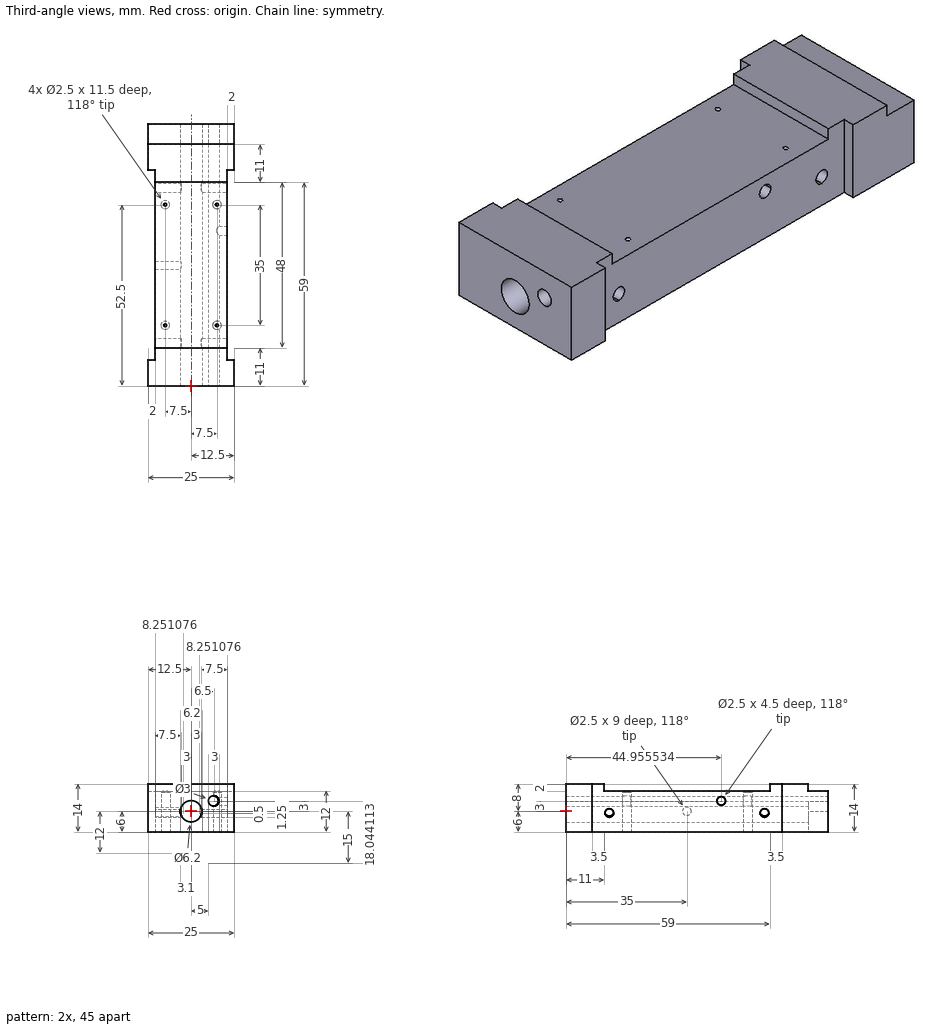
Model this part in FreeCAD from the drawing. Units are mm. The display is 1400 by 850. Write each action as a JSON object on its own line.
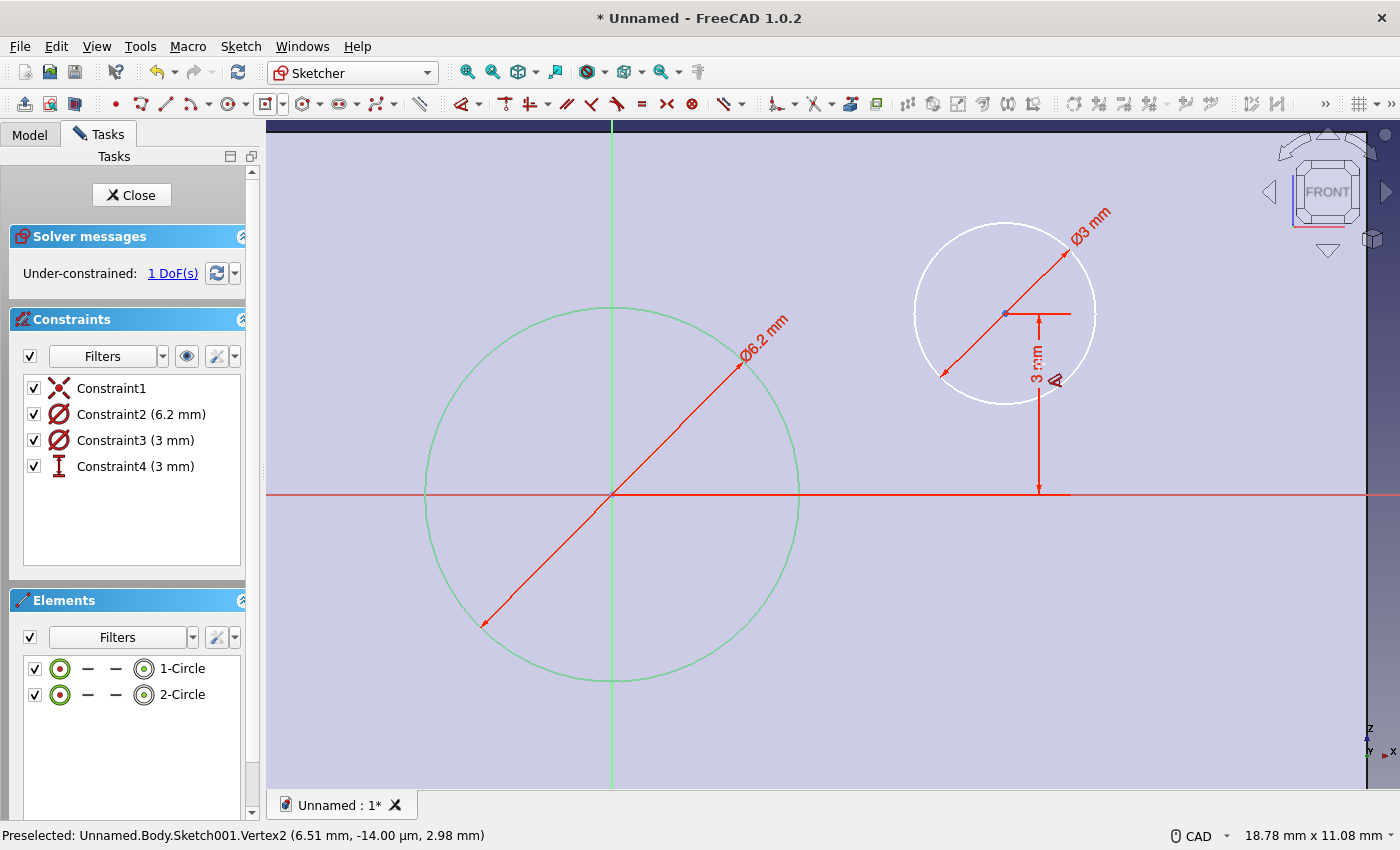
{"action": "left_click", "coordinate": [1005, 314]}
{"action": "left_click", "coordinate": [809, 280]}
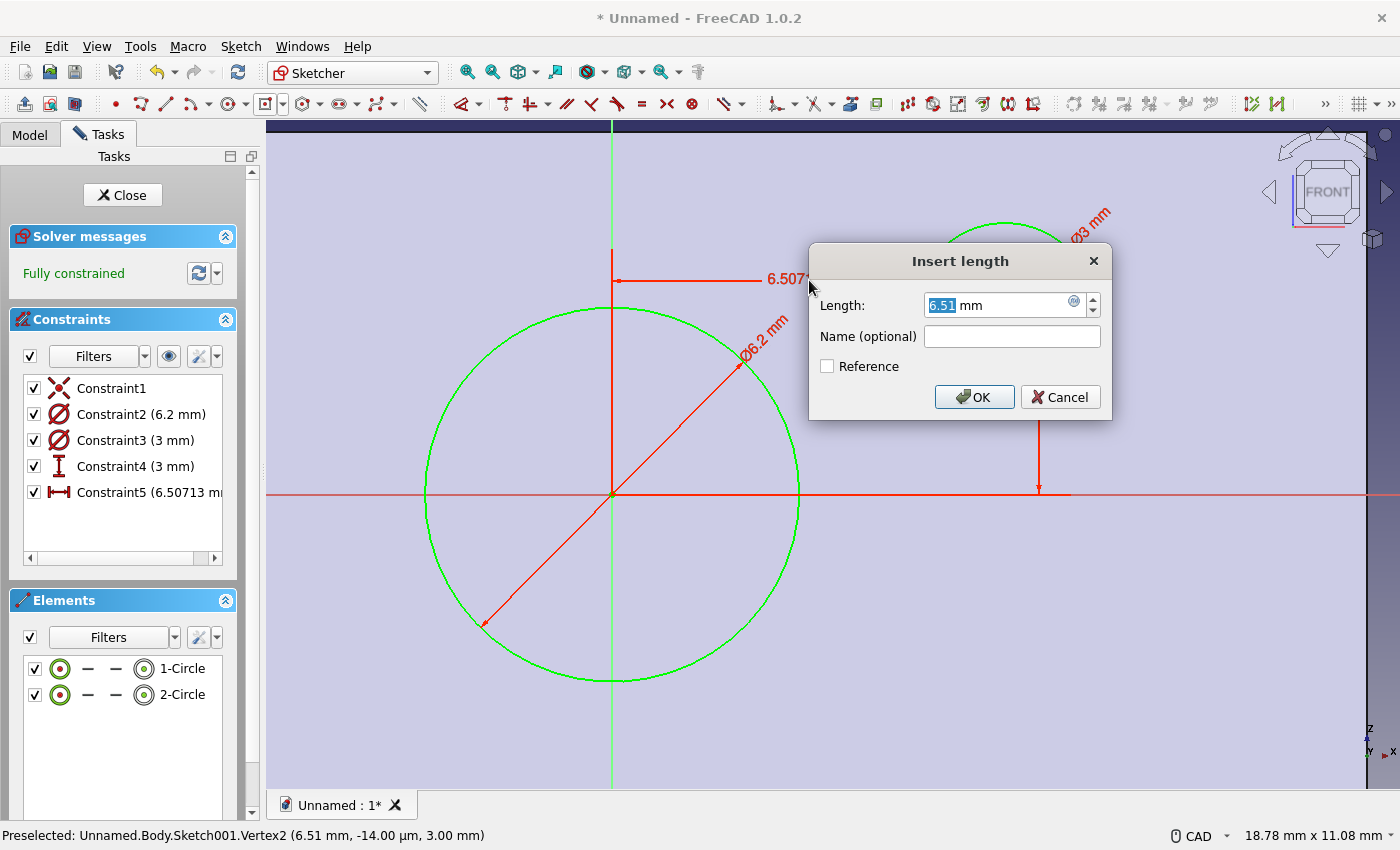
{"action": "type", "text": "6.5"}
{"action": "key", "text": "Return"}
{"action": "key", "text": "Escape"}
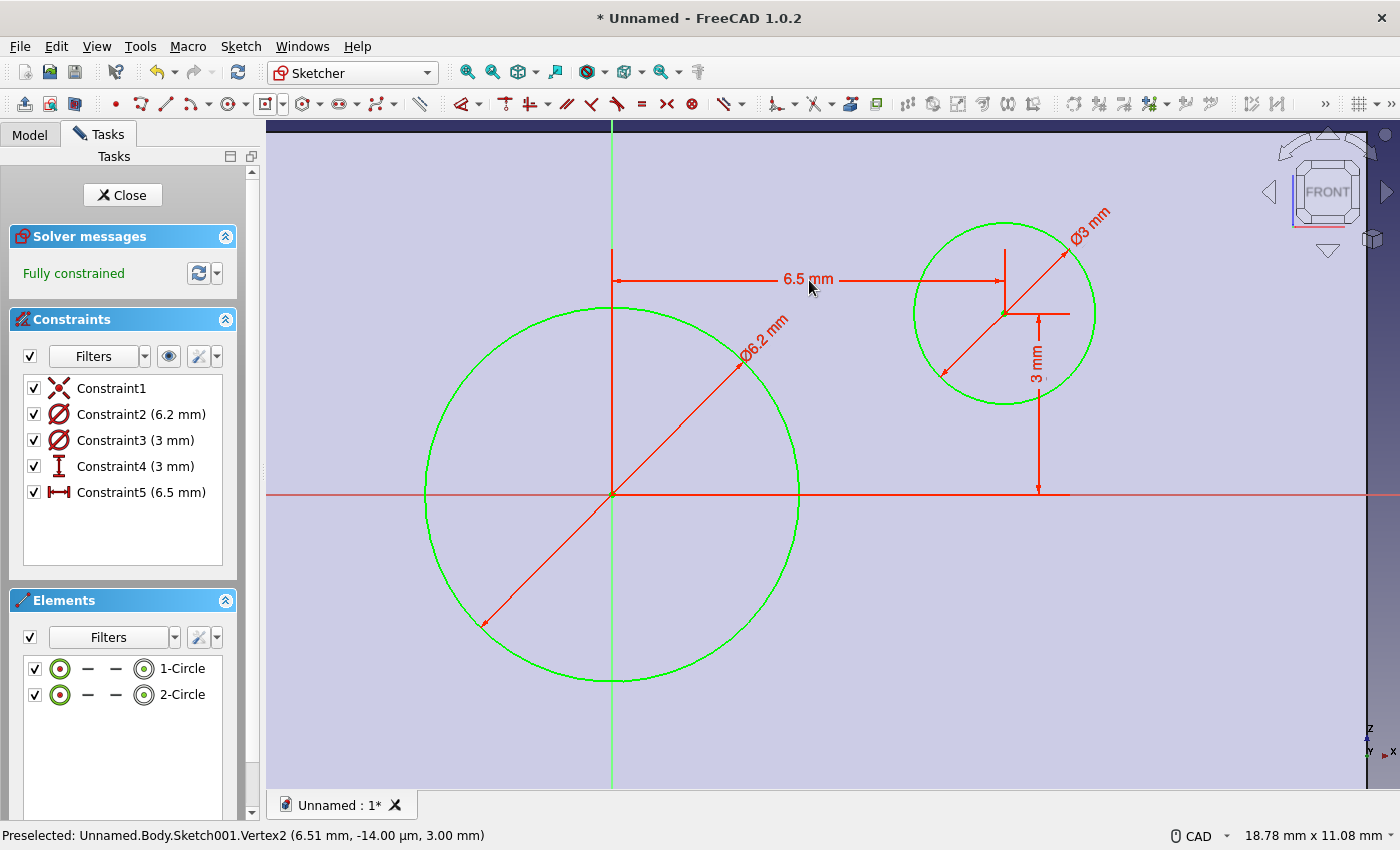
{"action": "left_click", "coordinate": [123, 195]}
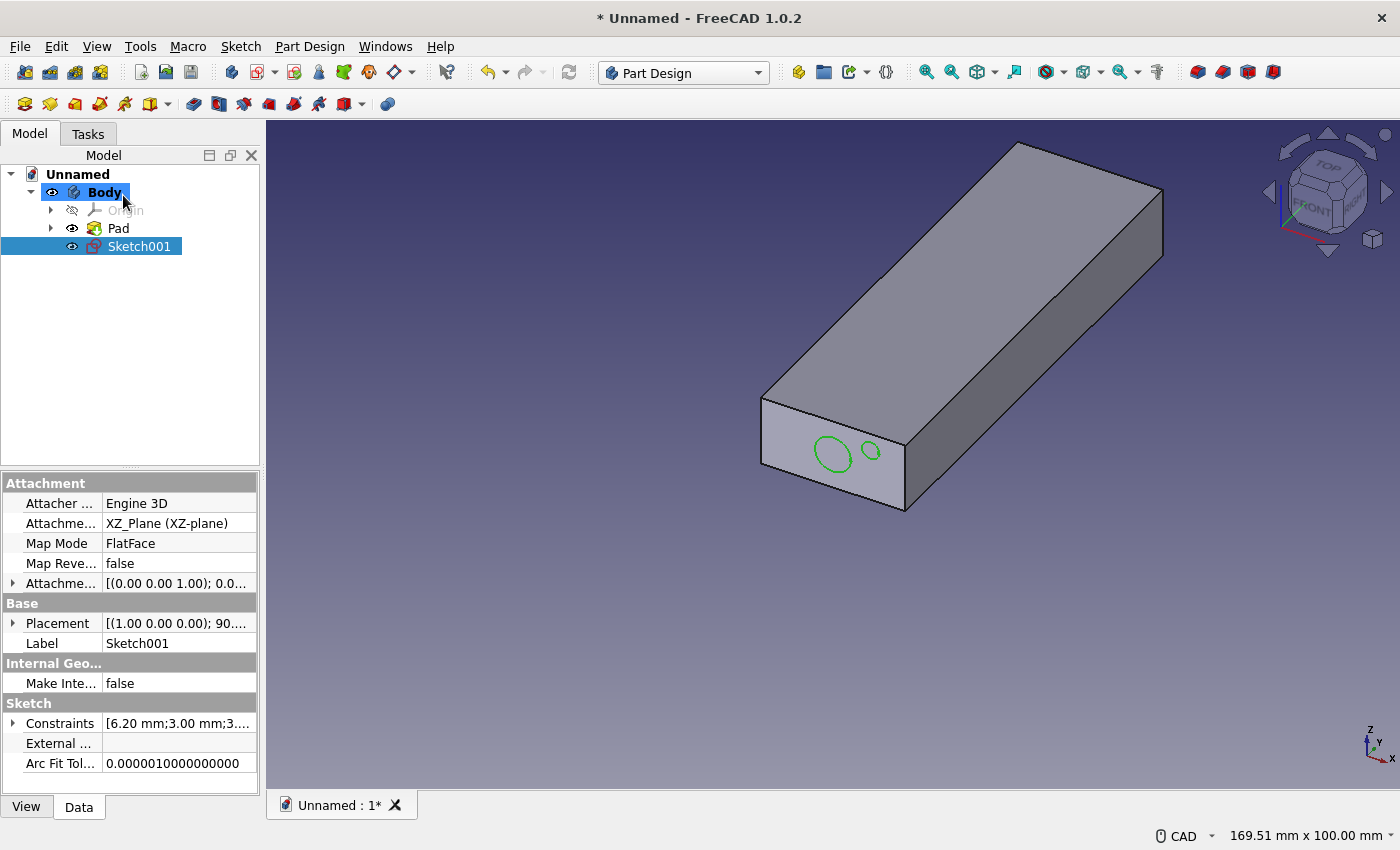
{"action": "left_click", "coordinate": [194, 104]}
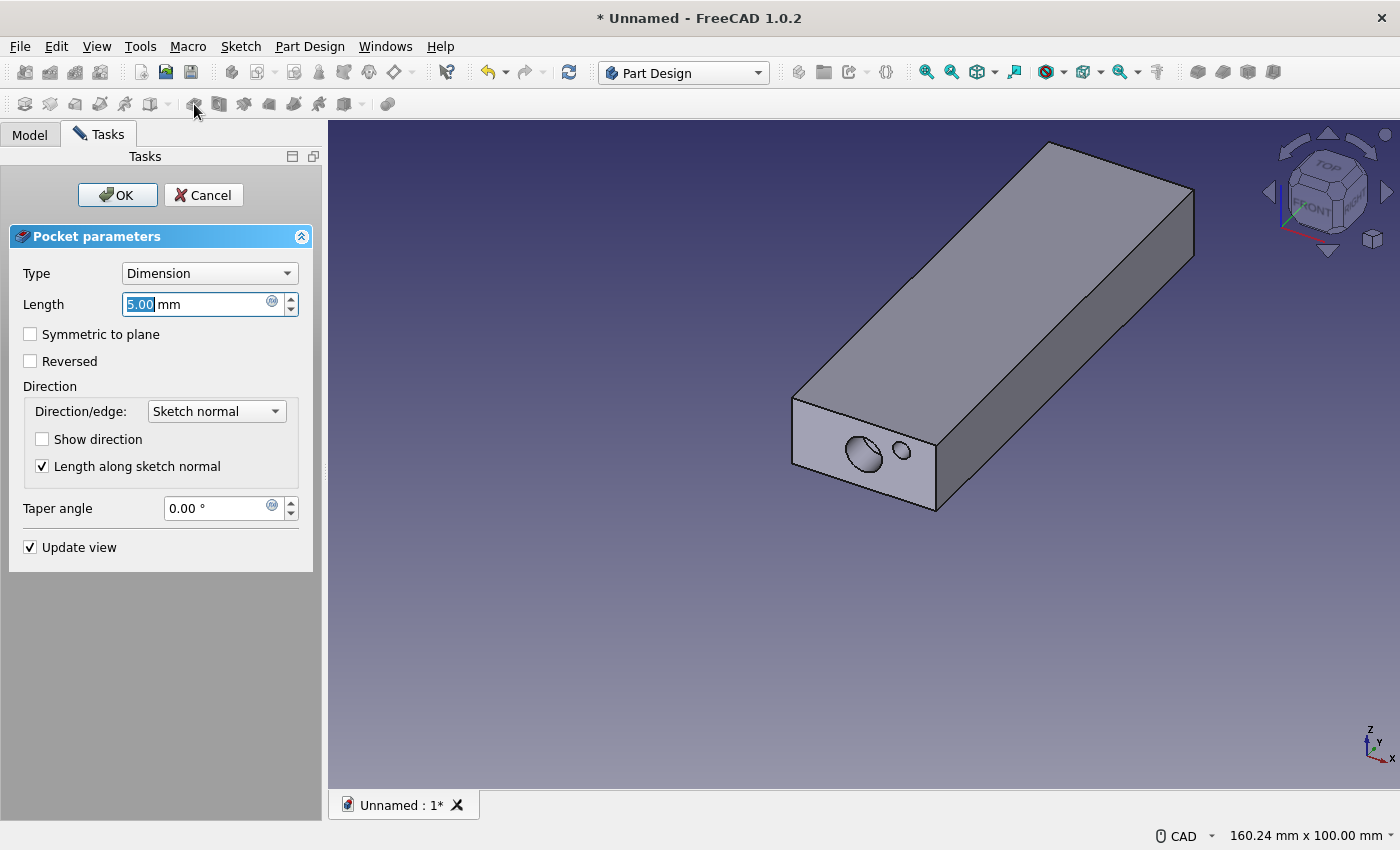
{"action": "left_click", "coordinate": [210, 274]}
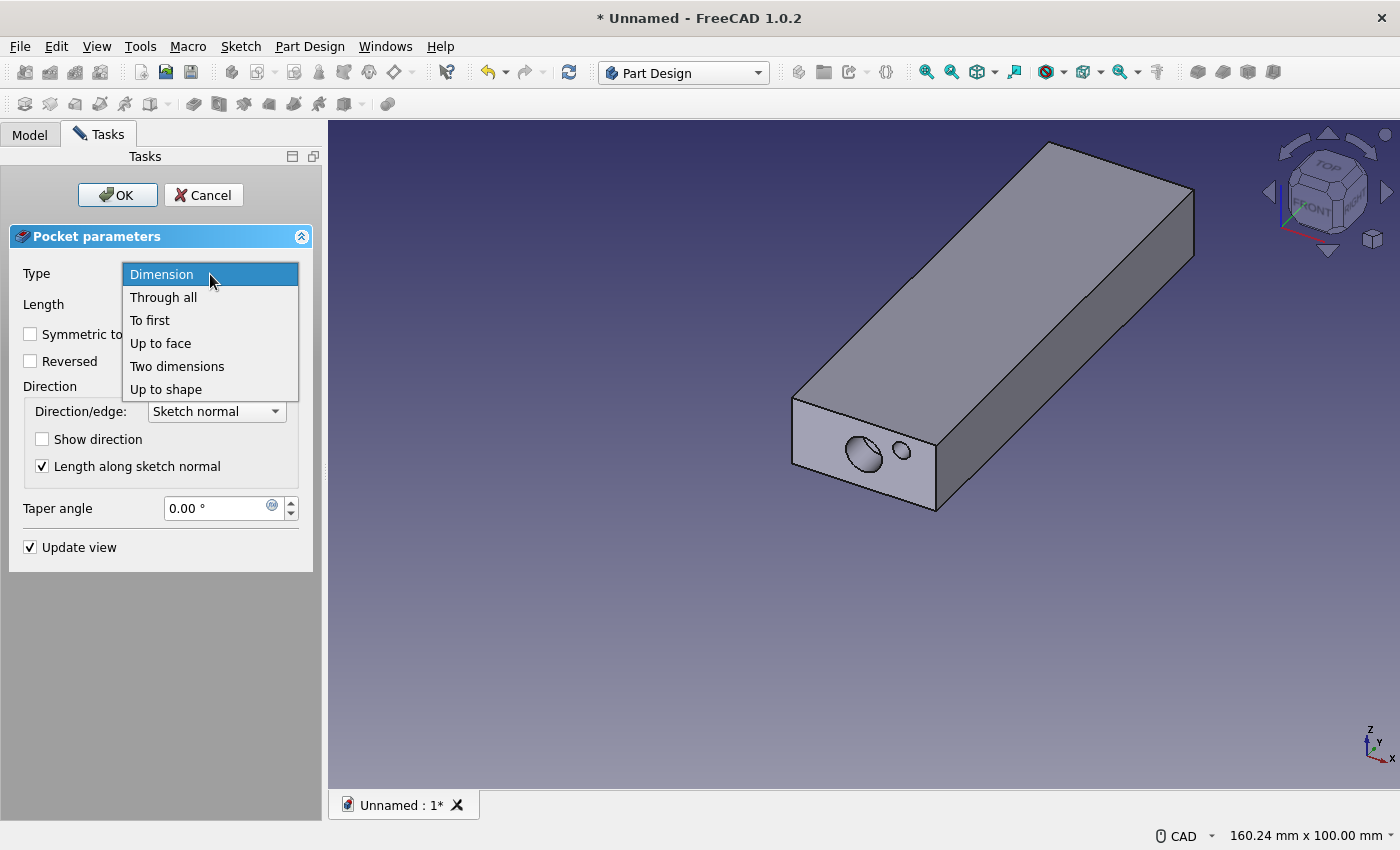
{"action": "left_click", "coordinate": [208, 298]}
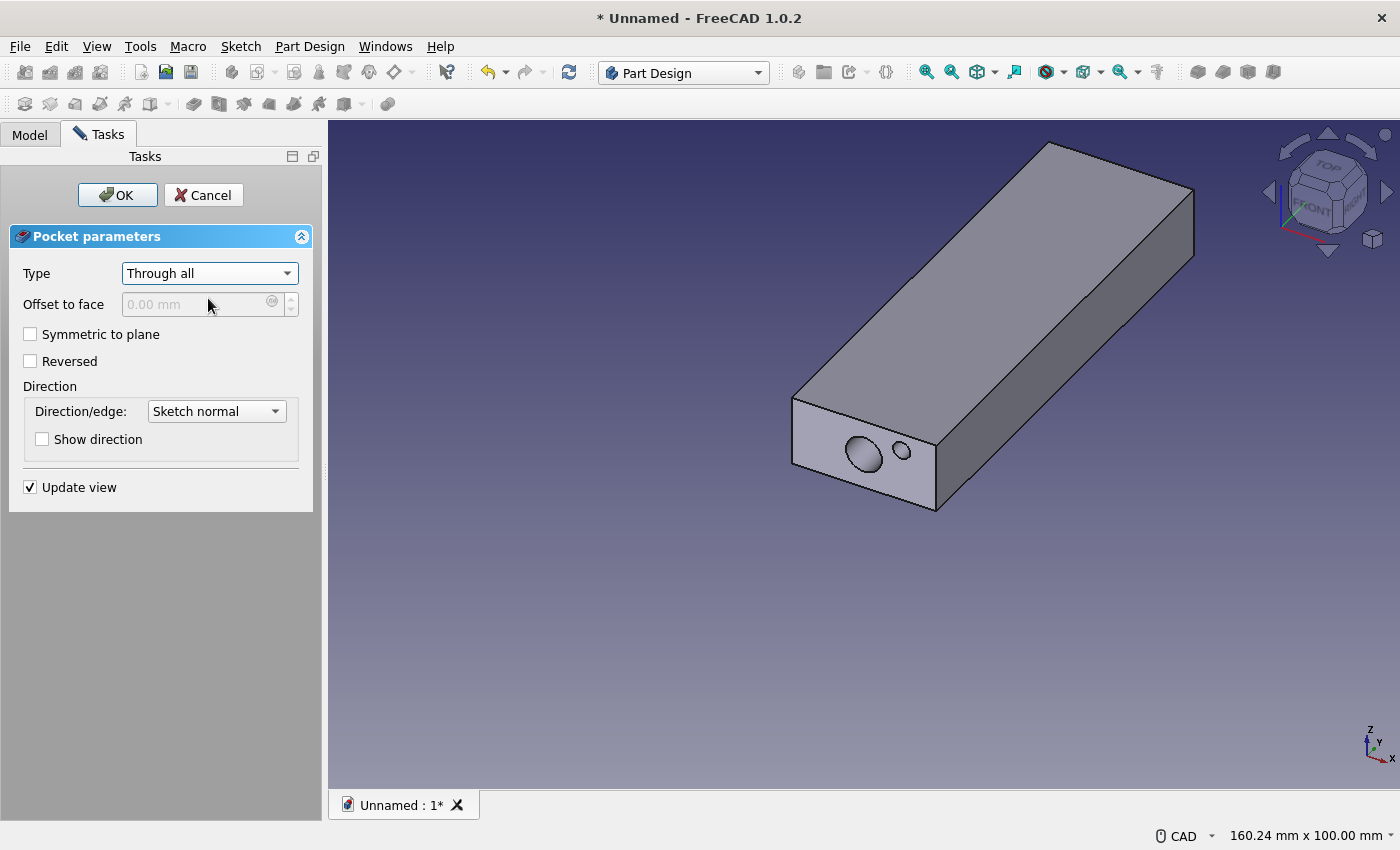
{"action": "left_click", "coordinate": [118, 195]}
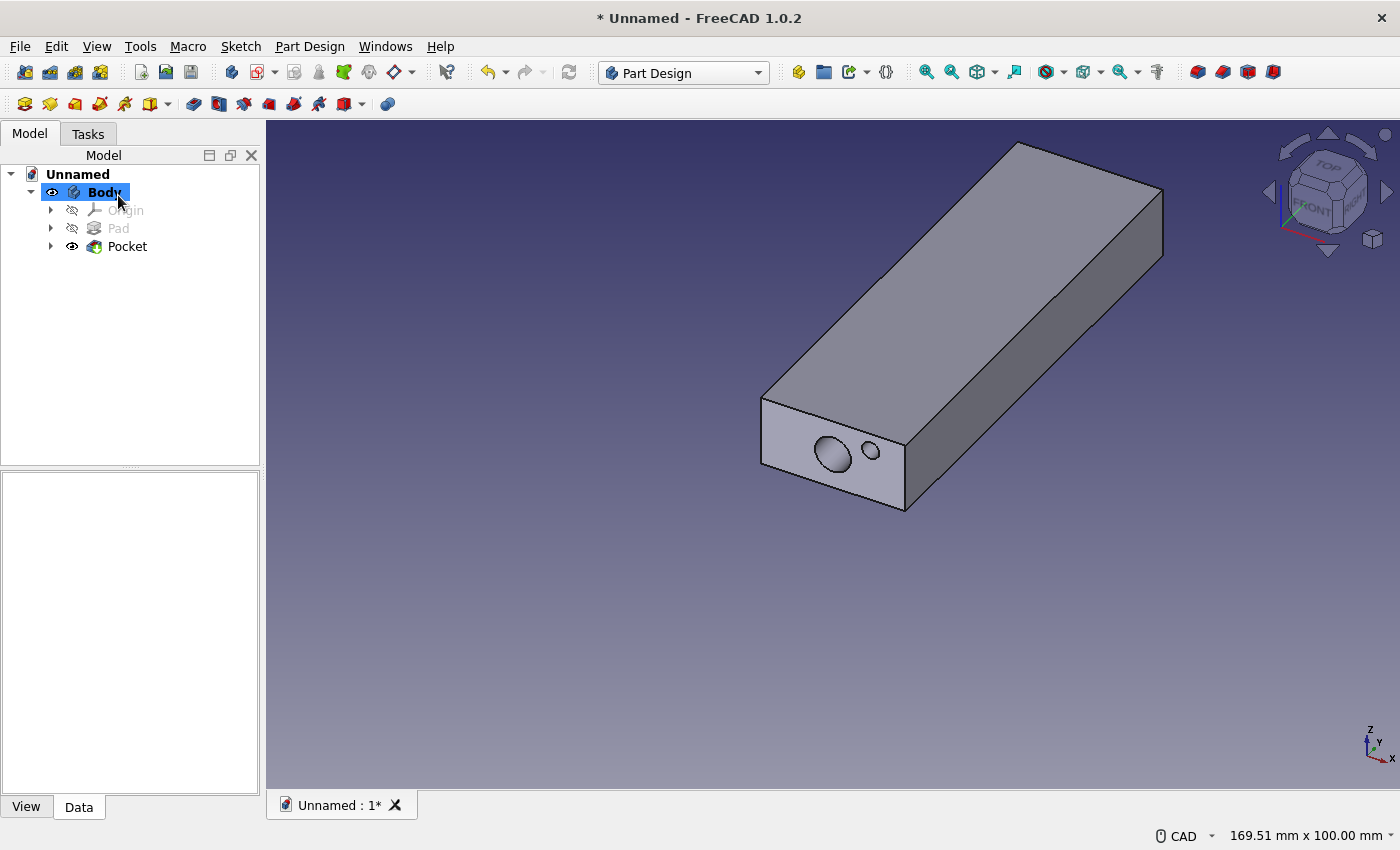
{"action": "key", "text": "4"}